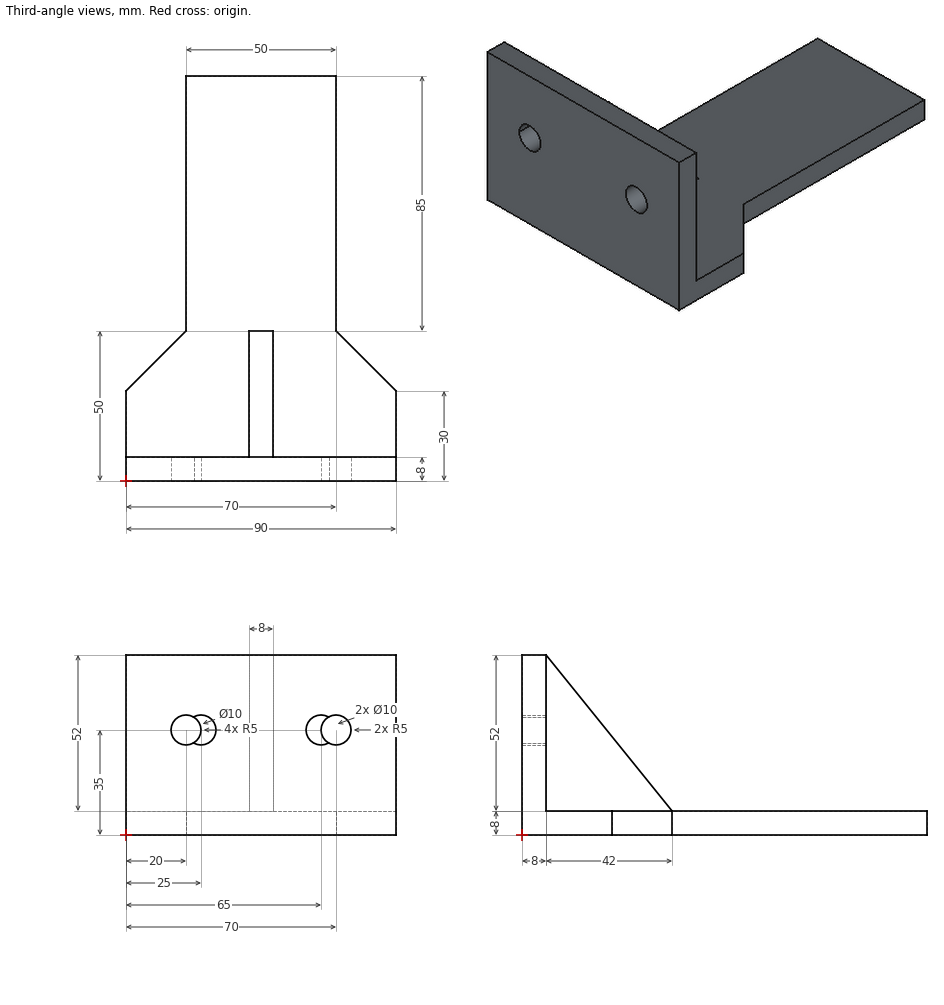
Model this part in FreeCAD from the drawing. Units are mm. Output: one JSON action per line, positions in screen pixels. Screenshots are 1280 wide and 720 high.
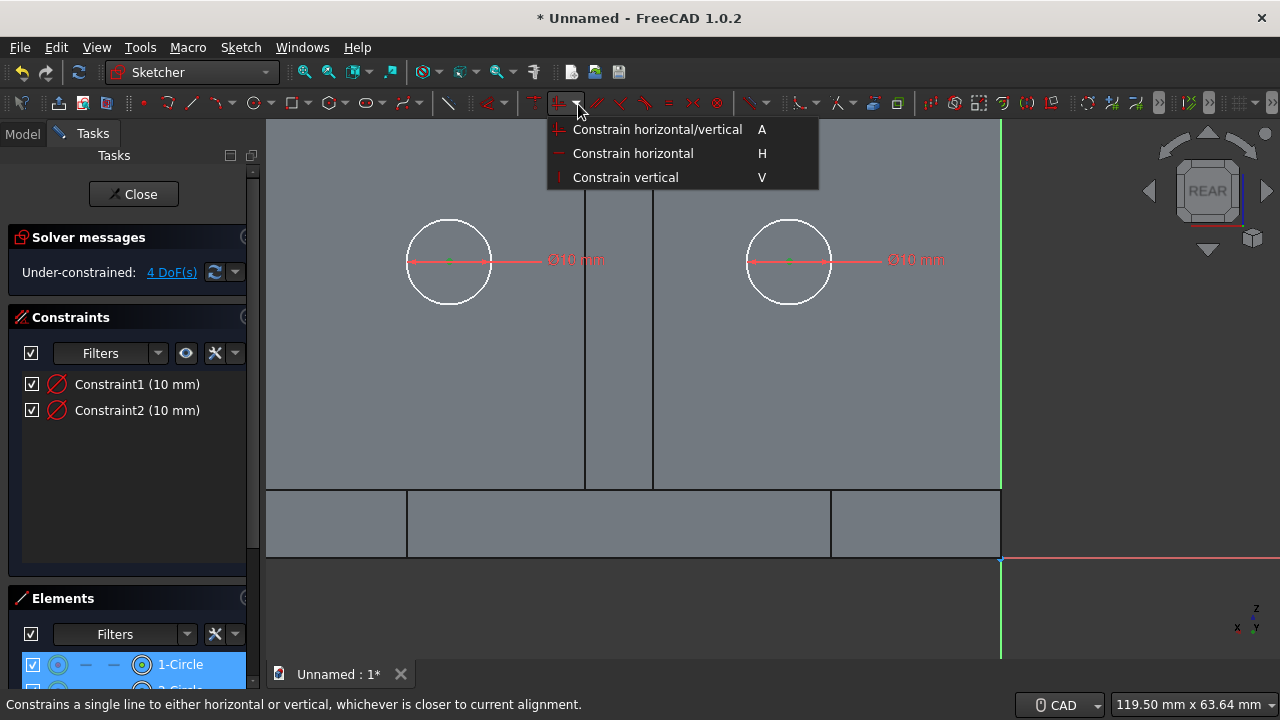
{"action": "left_click", "coordinate": [683, 153]}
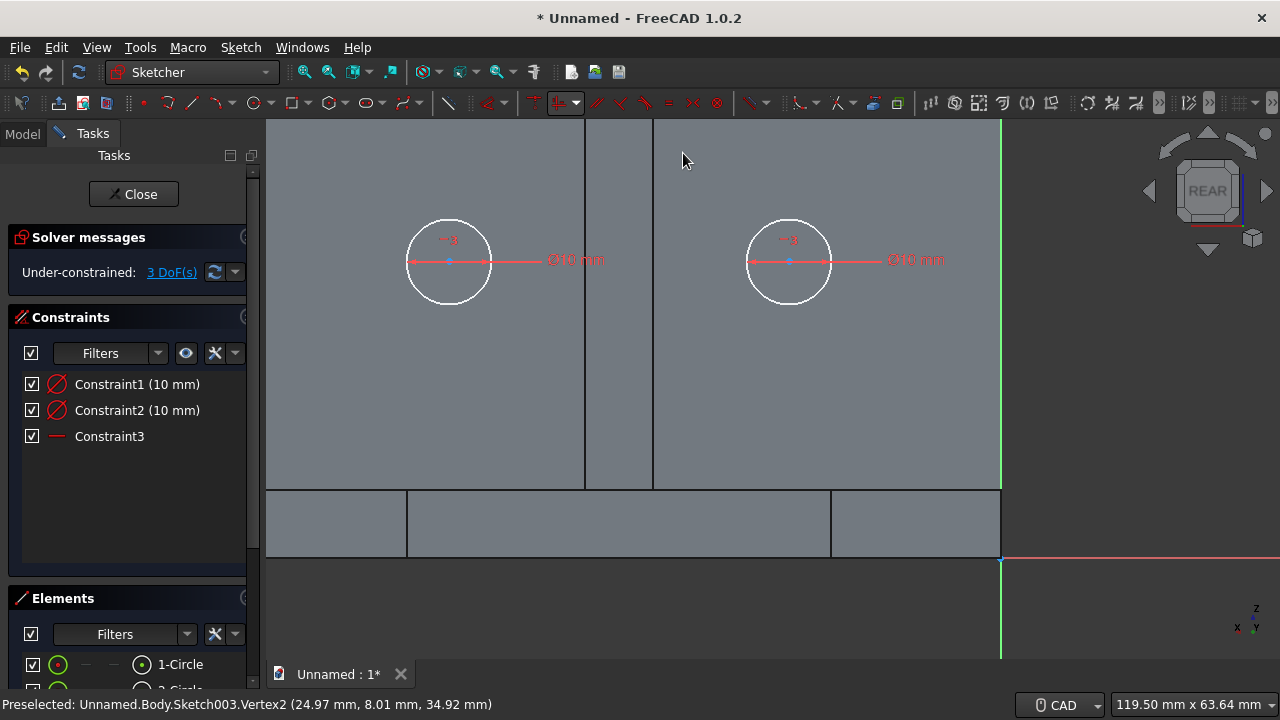
{"action": "left_click", "coordinate": [488, 104]}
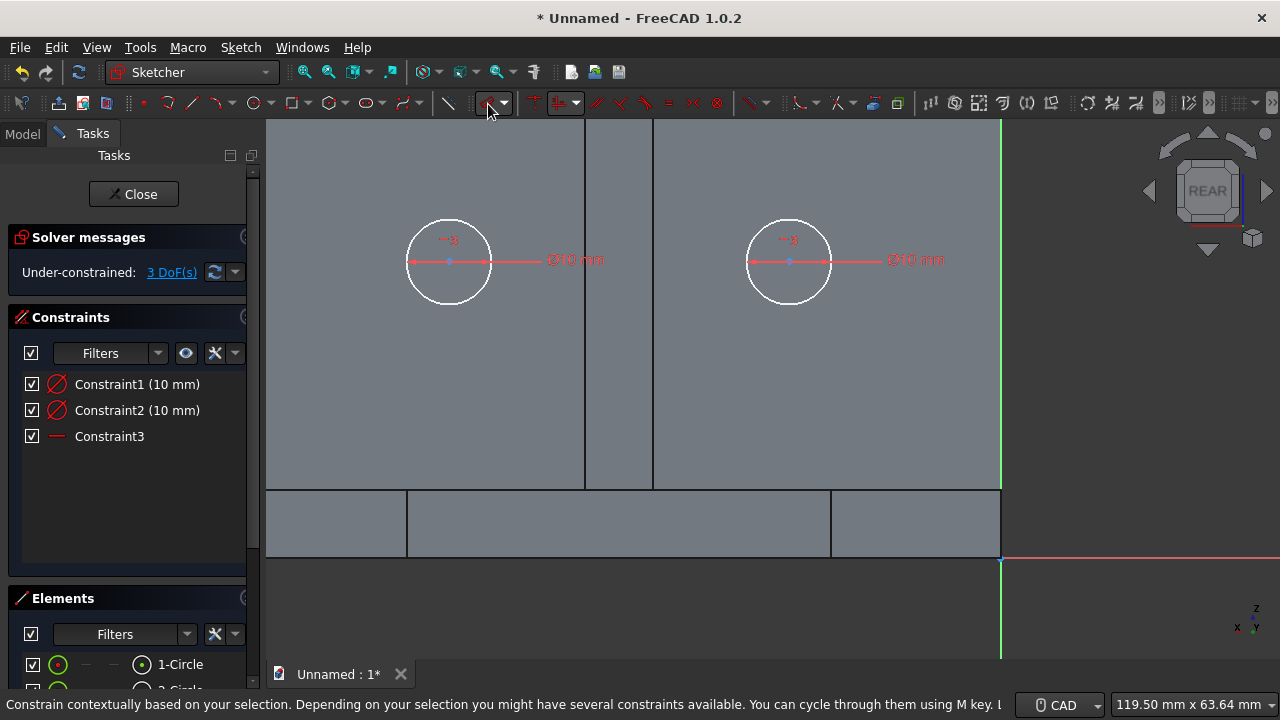
{"action": "left_click", "coordinate": [449, 262]}
{"action": "left_click", "coordinate": [725, 592]}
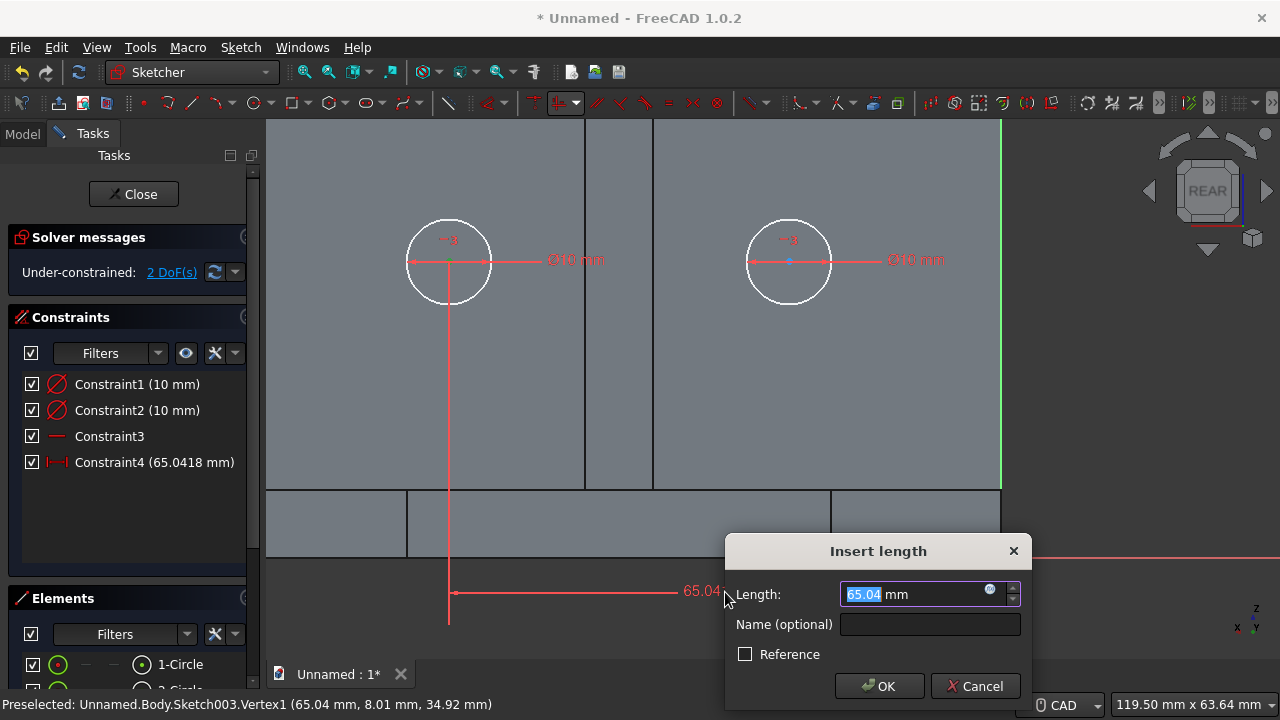
{"action": "type", "text": "65"}
{"action": "key", "text": "Return"}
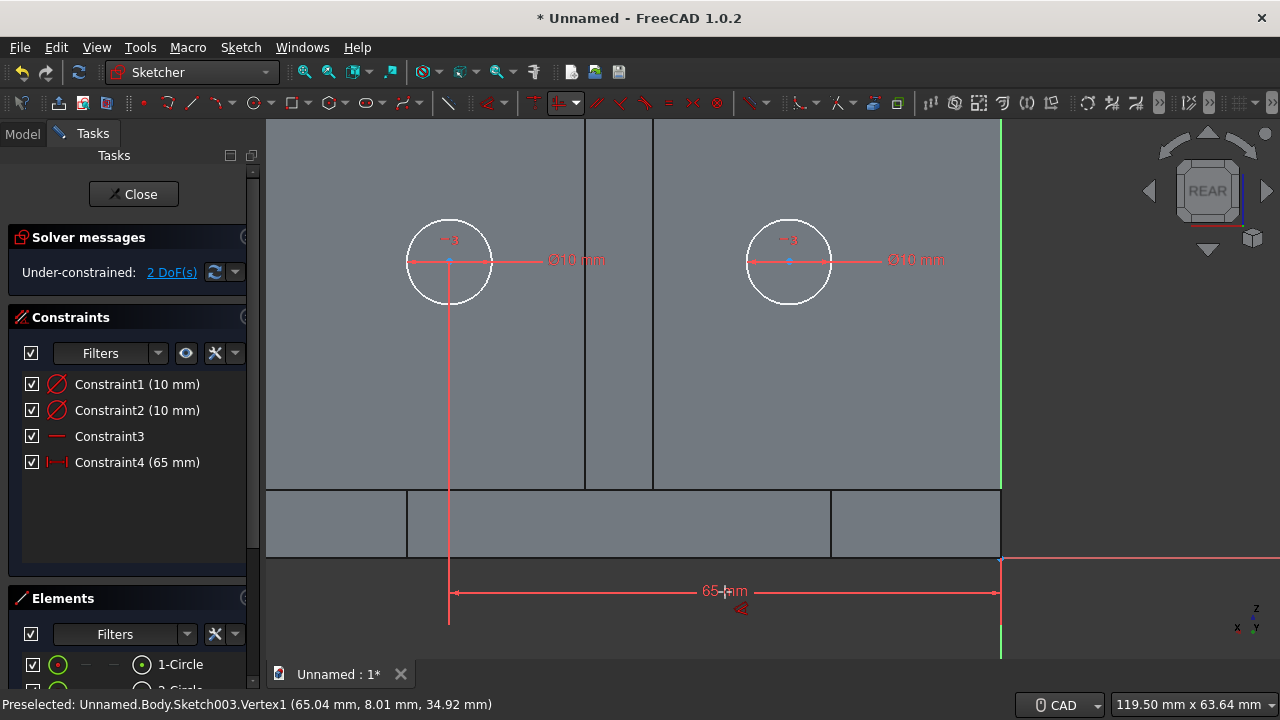
{"action": "left_click", "coordinate": [449, 262]}
{"action": "left_click", "coordinate": [1035, 410]}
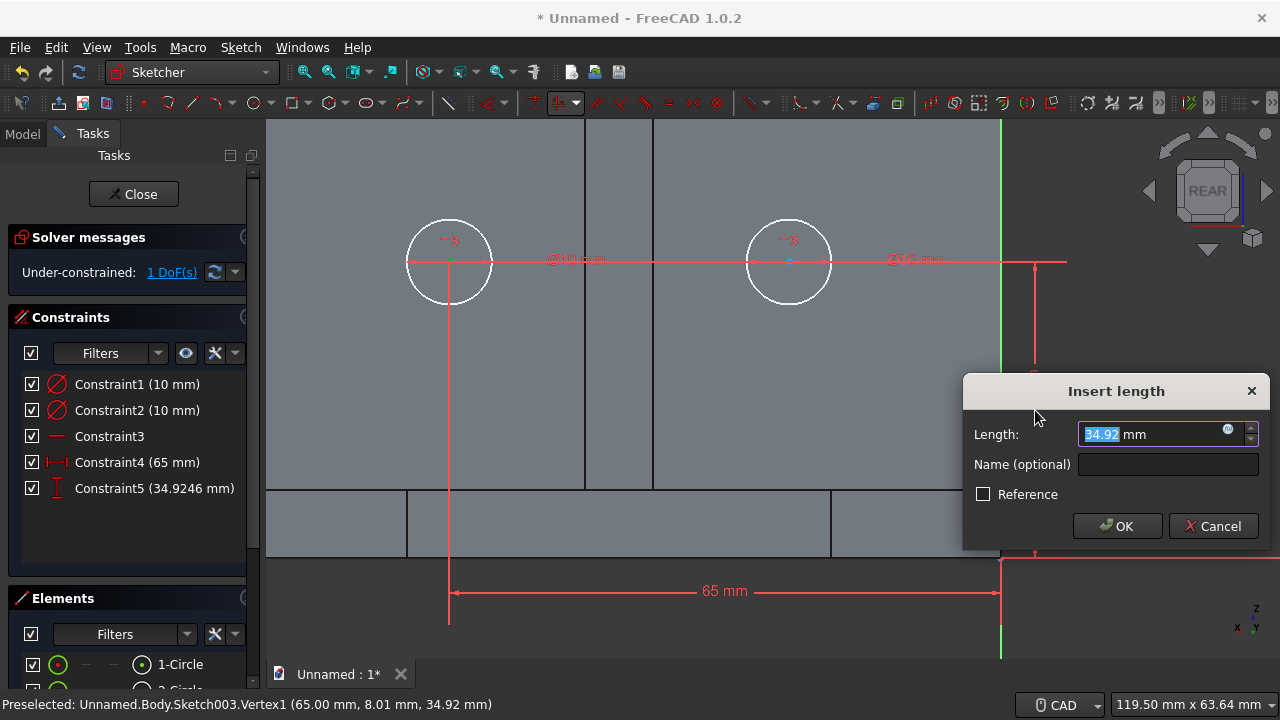
{"action": "type", "text": "35"}
{"action": "key", "text": "Return"}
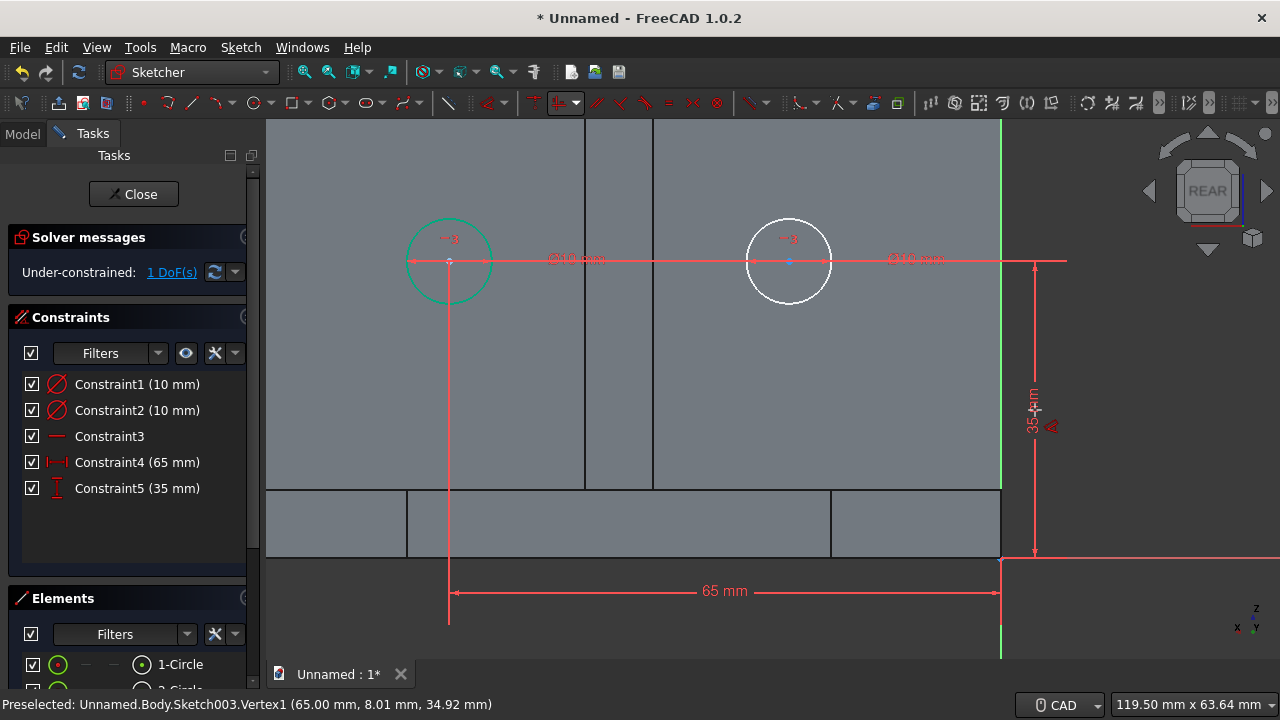
{"action": "left_click", "coordinate": [789, 261]}
{"action": "left_click", "coordinate": [895, 592]}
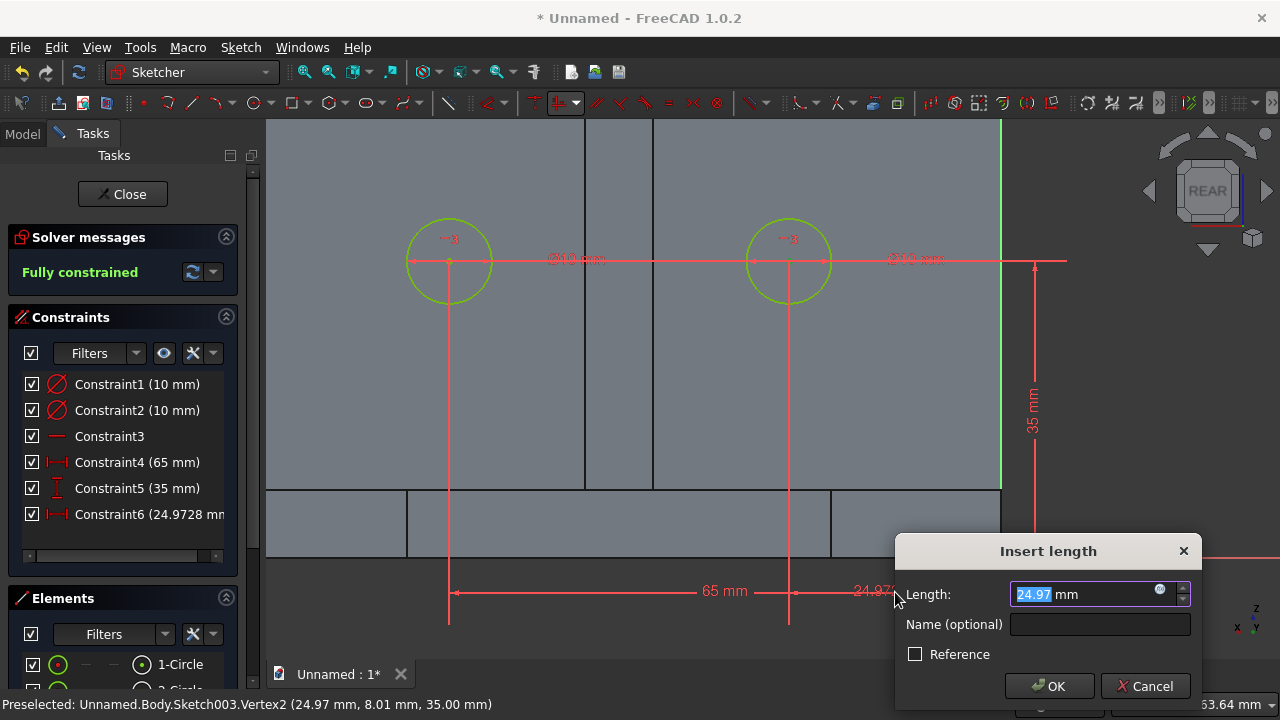
{"action": "type", "text": "25"}
{"action": "key", "text": "Return"}
{"action": "key", "text": "Escape"}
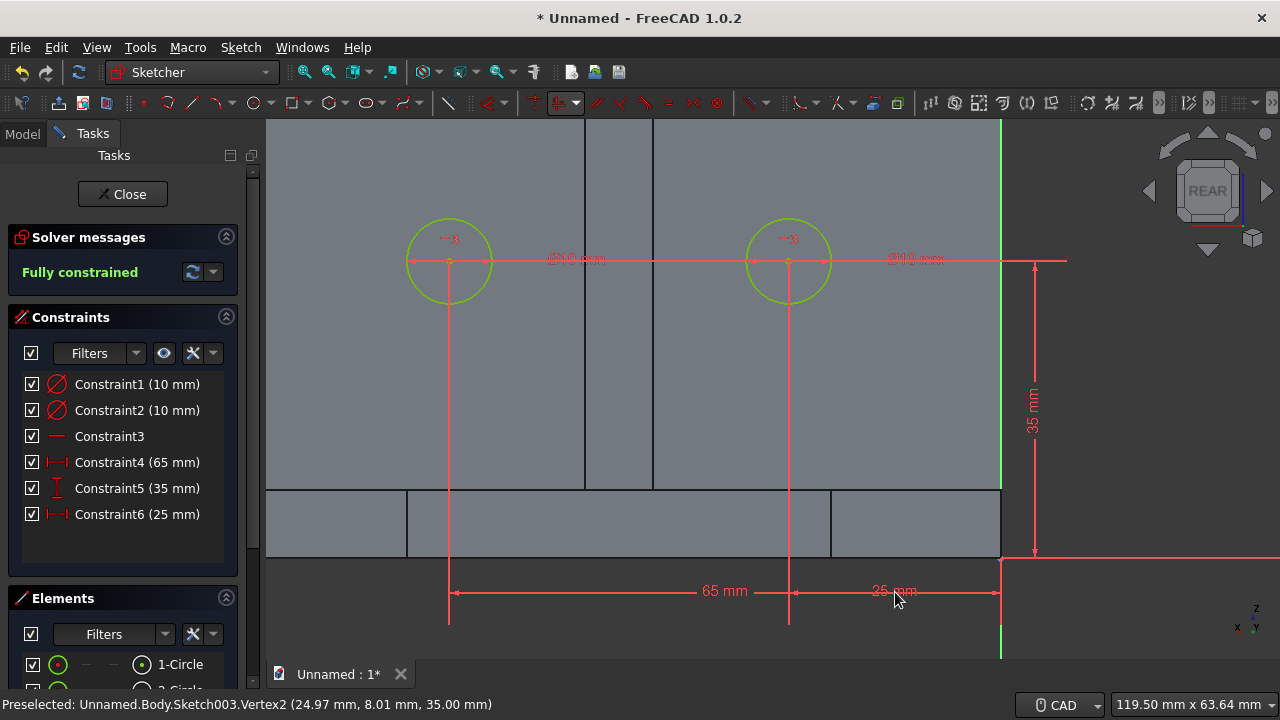
{"action": "left_click", "coordinate": [123, 194]}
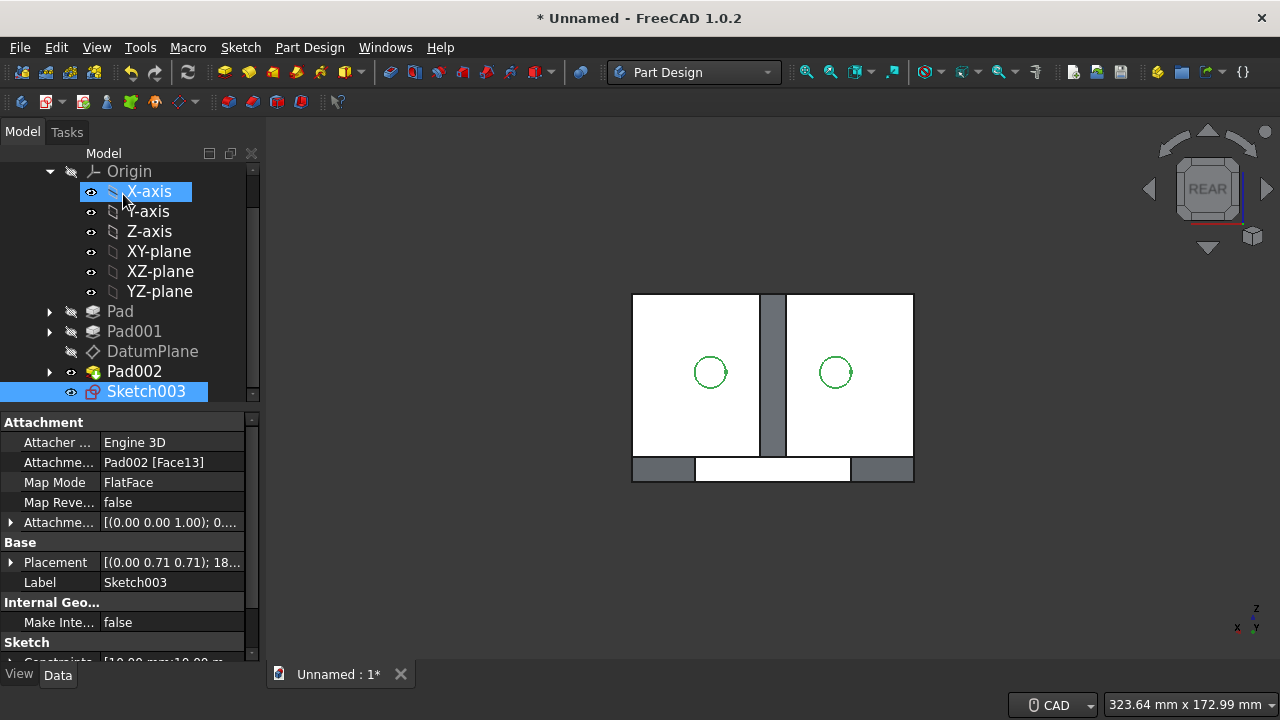
{"action": "left_click", "coordinate": [392, 72]}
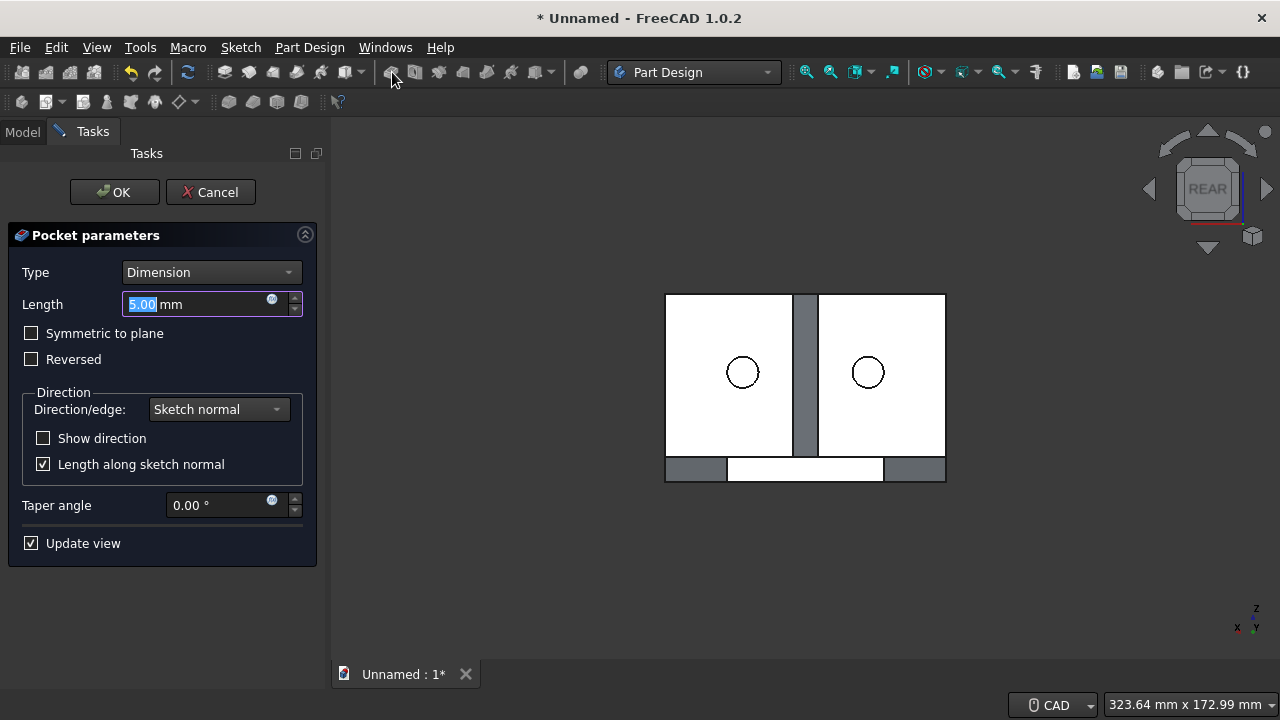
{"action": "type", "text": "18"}
{"action": "key", "text": "Tab"}